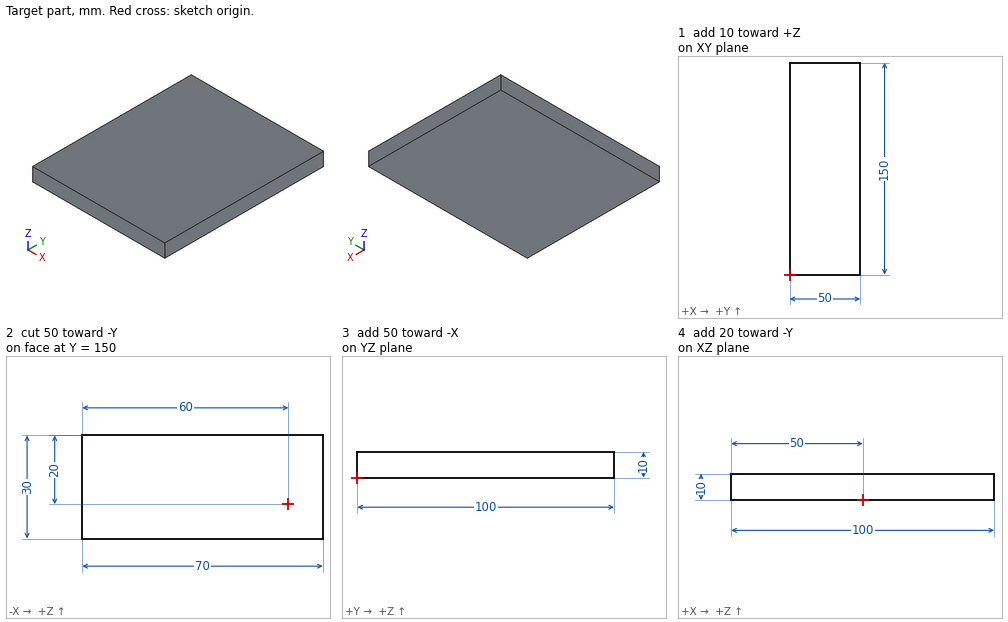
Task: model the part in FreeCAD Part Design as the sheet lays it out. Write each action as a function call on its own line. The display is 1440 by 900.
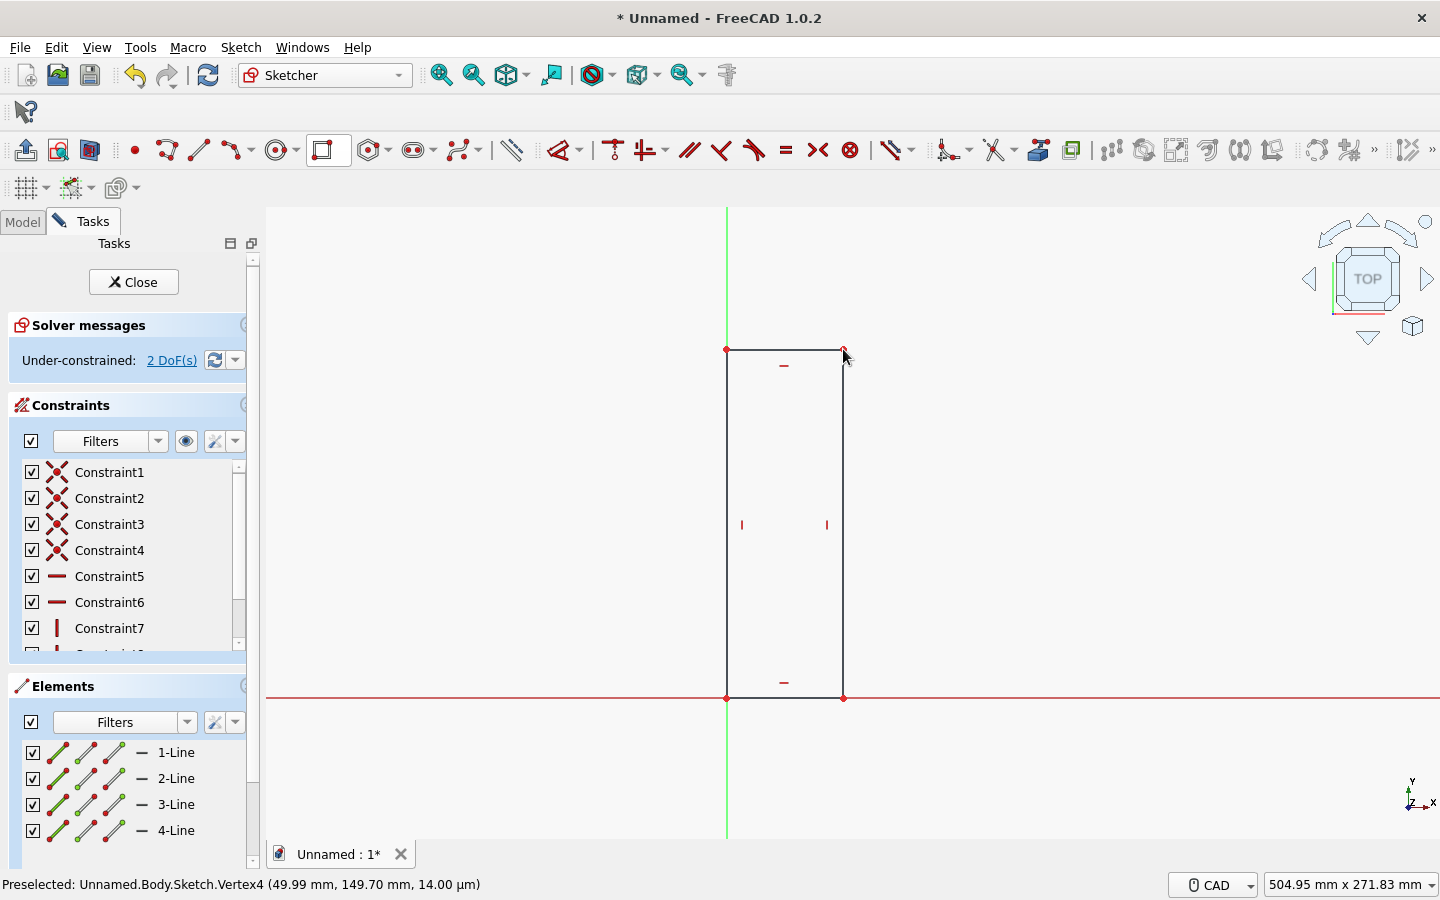
click(558, 150)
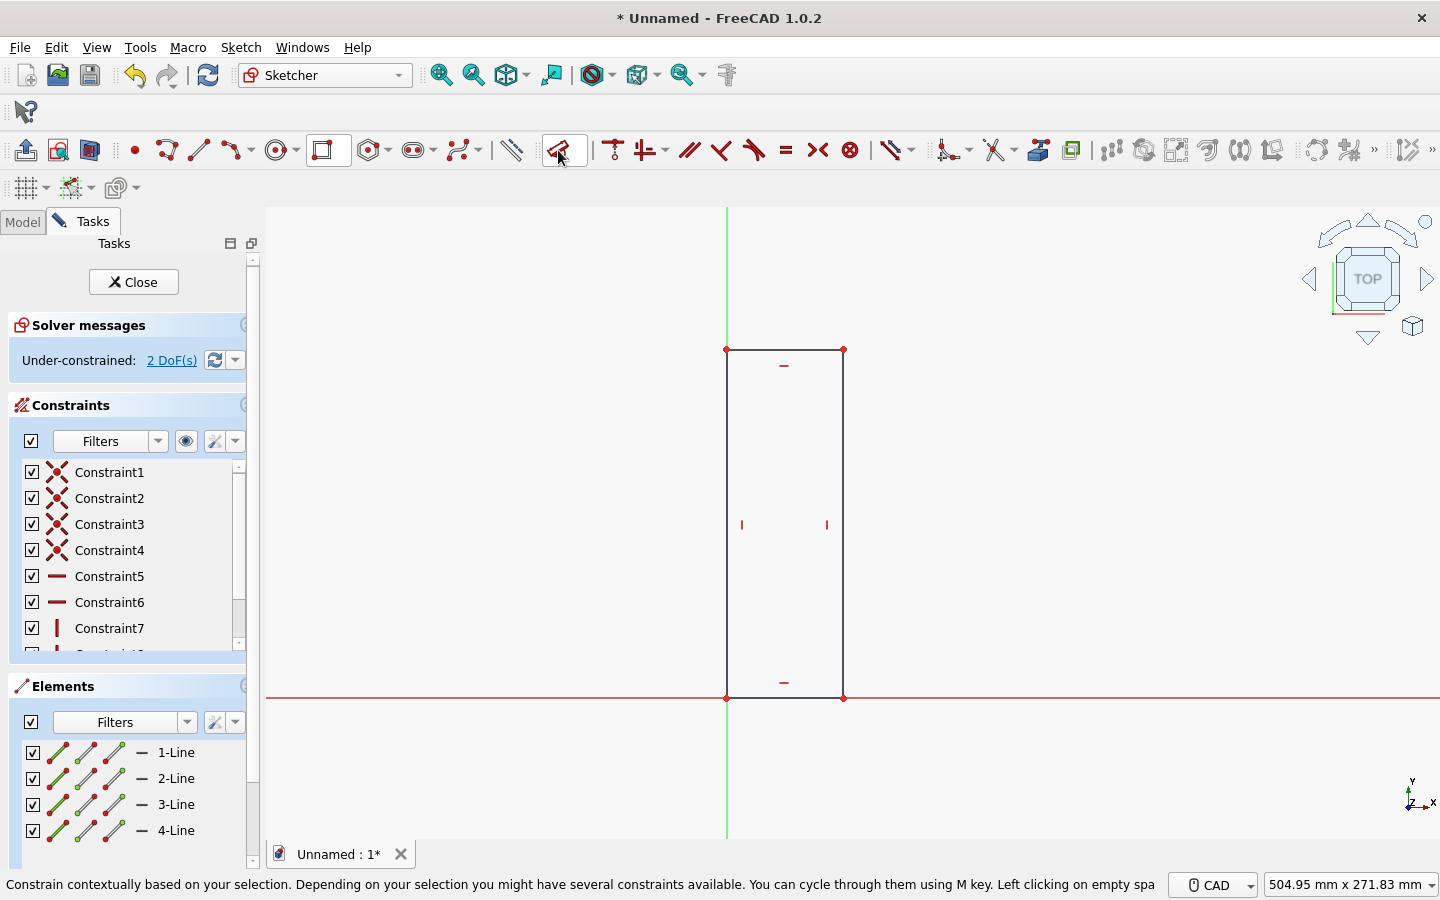
click(762, 698)
click(785, 732)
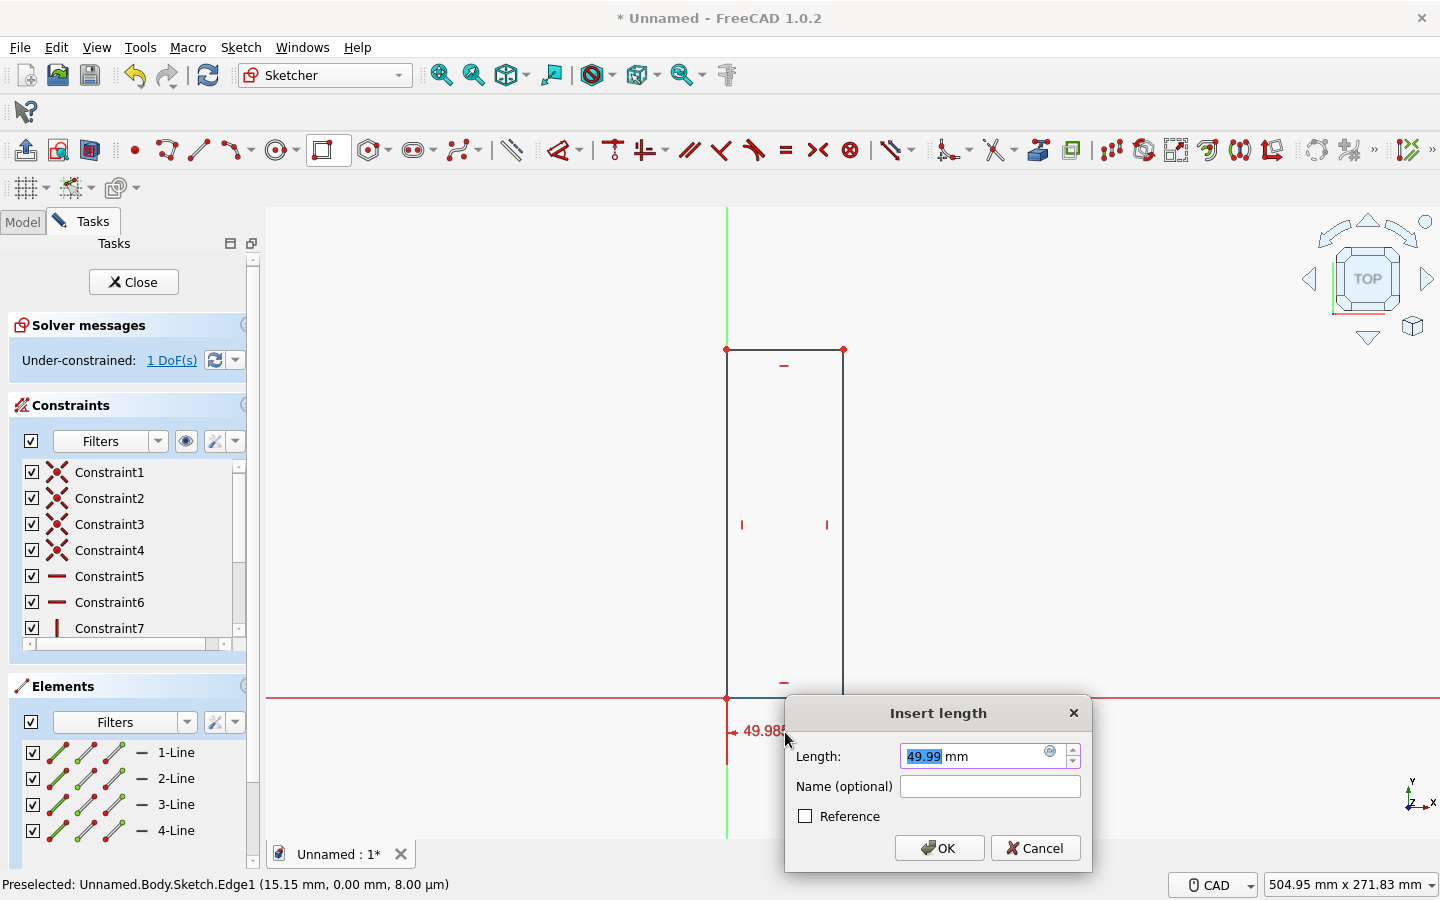
text(50)
key(Return)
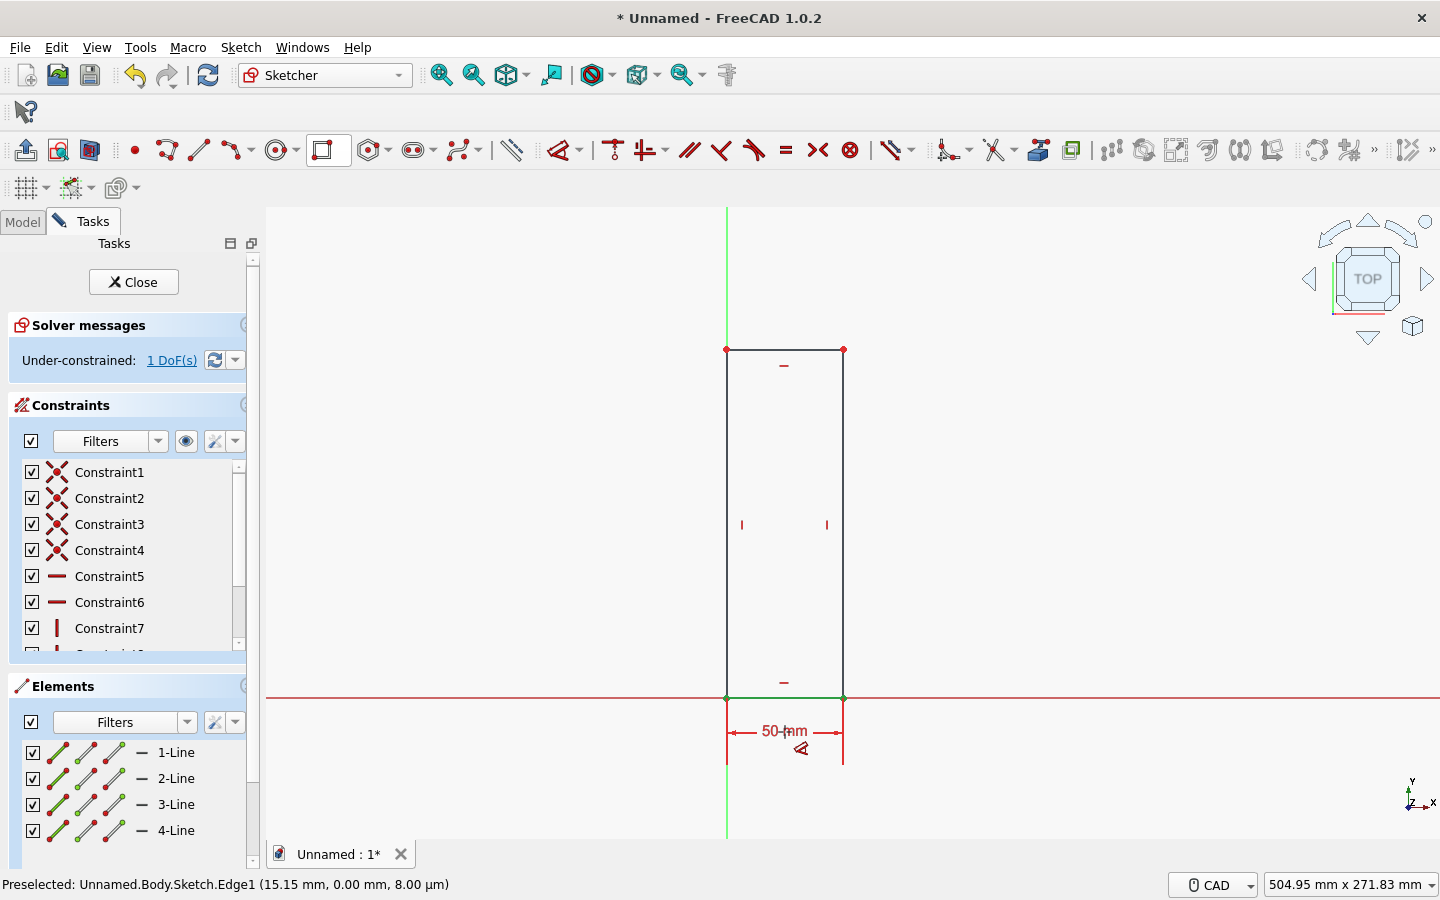
click(843, 594)
click(877, 524)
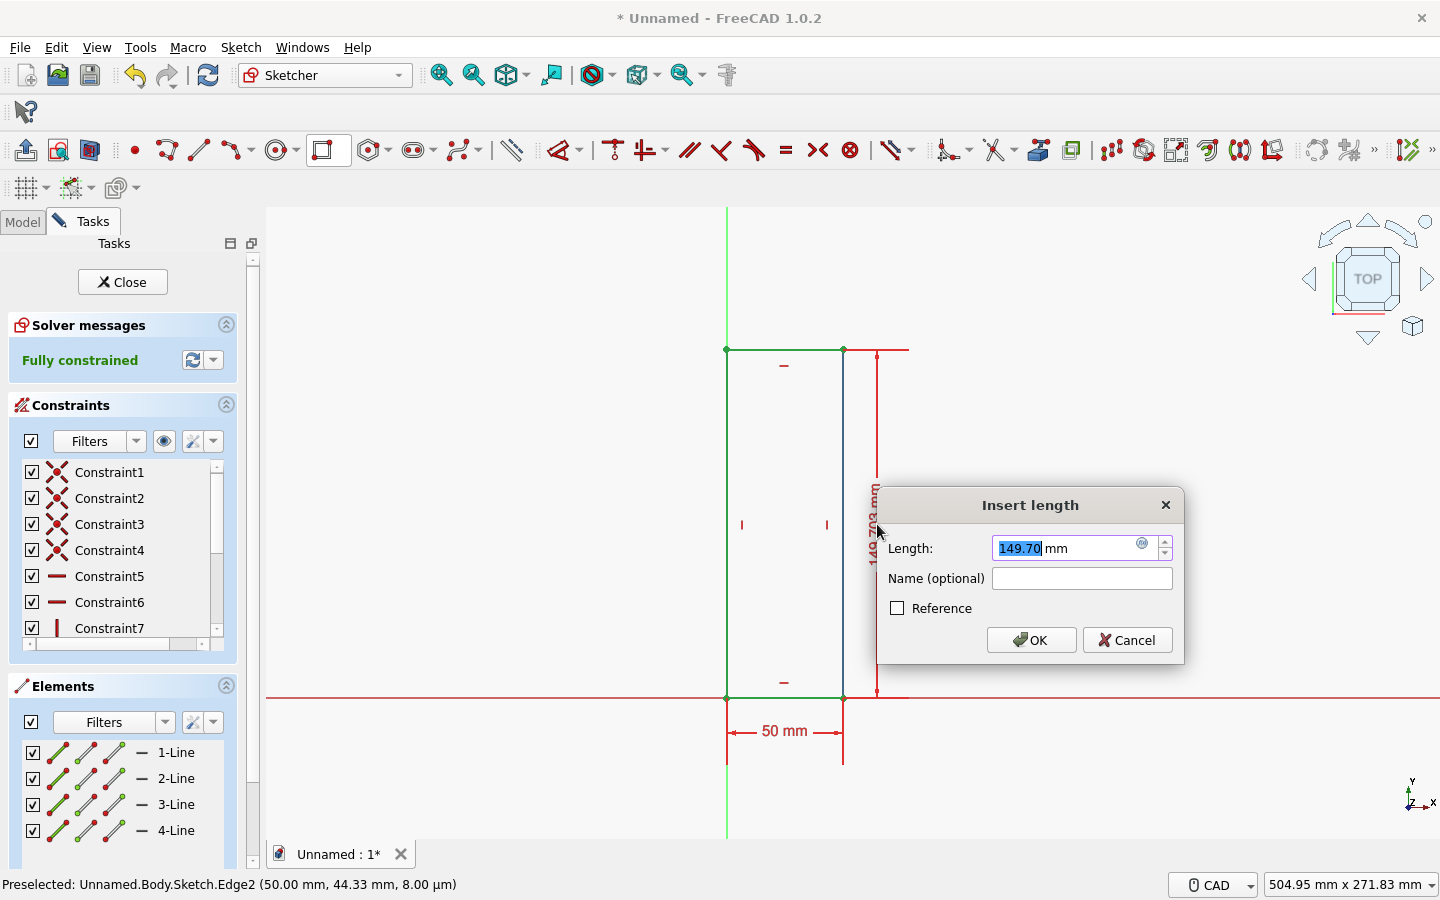
text(150)
key(Return)
key(Escape)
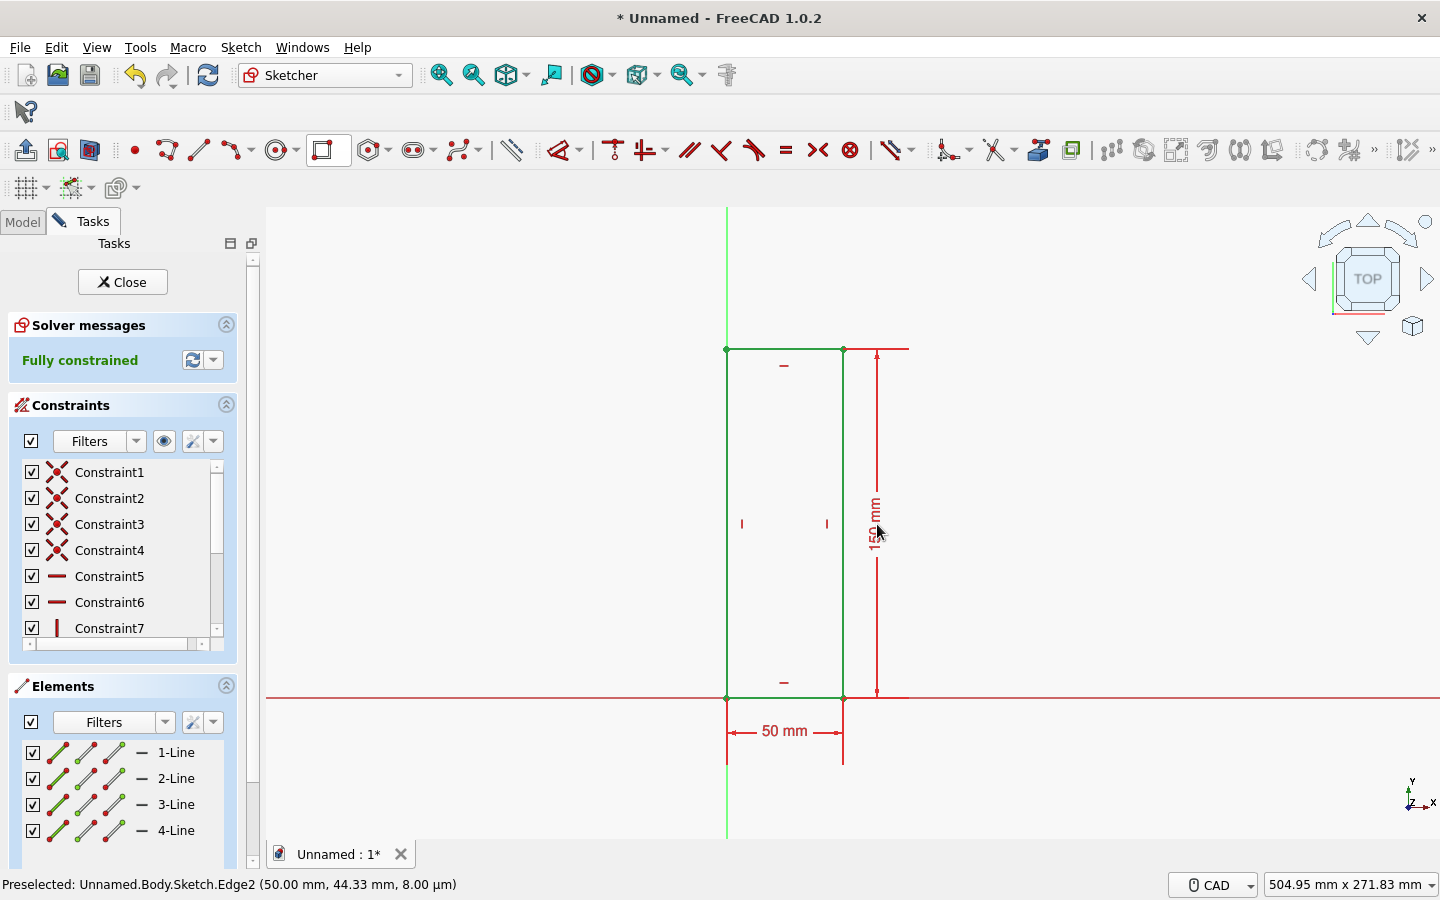
click(123, 282)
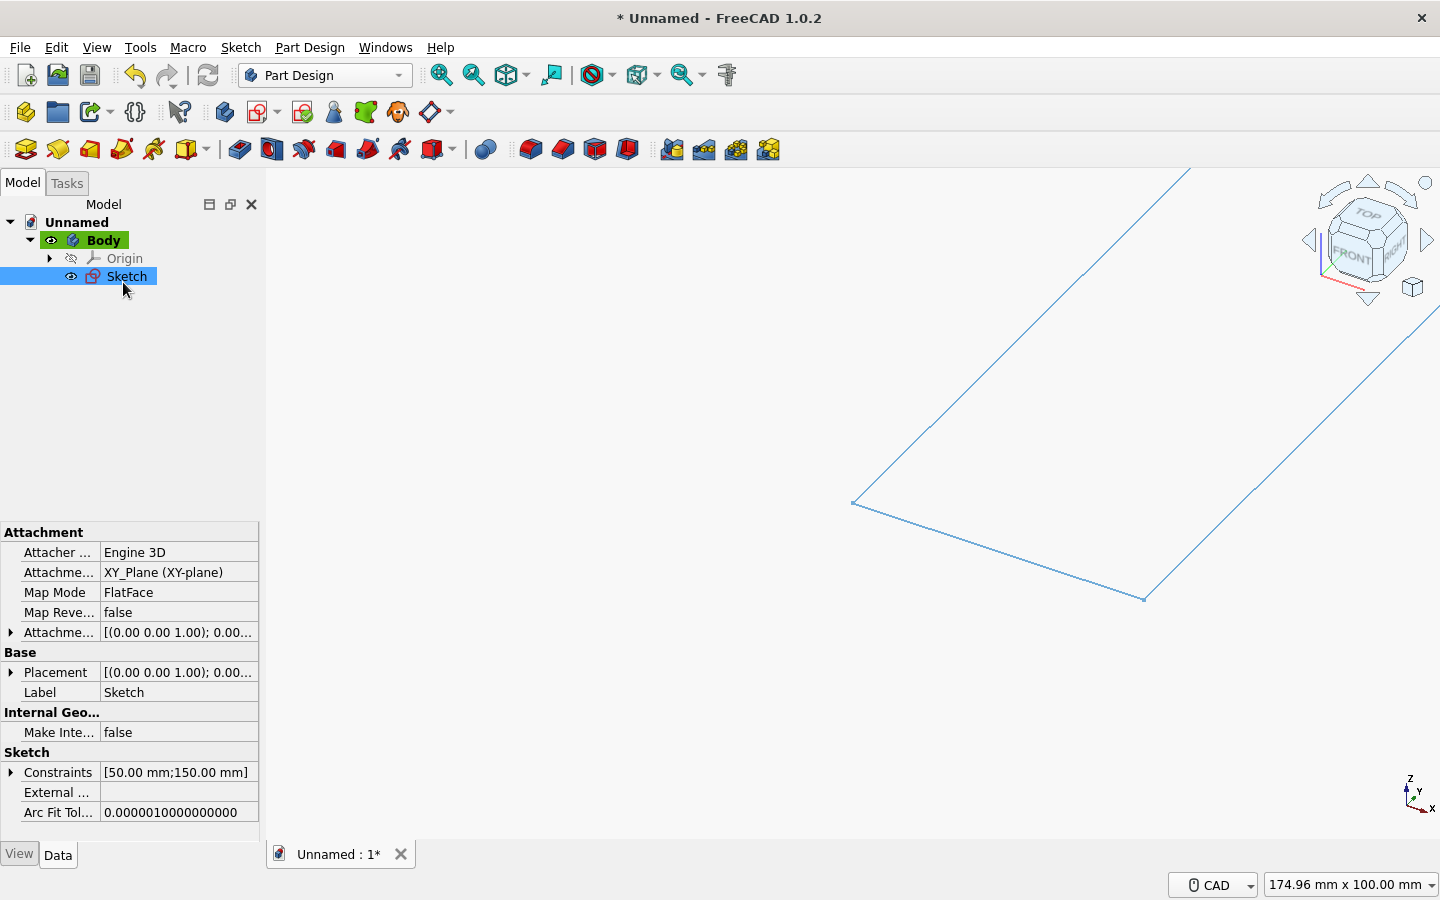
click(26, 150)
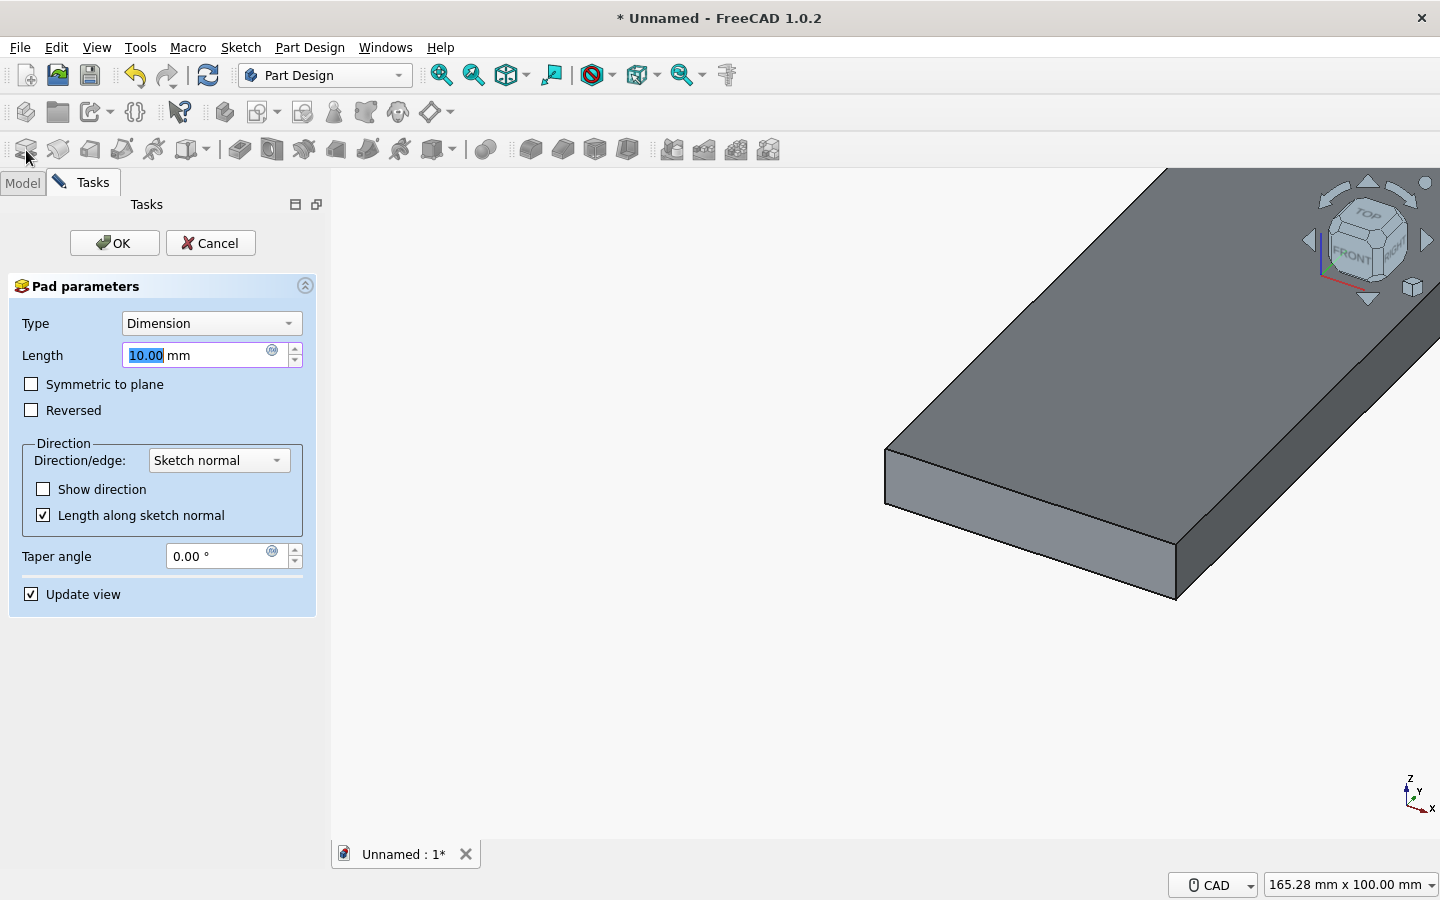
text(10)
key(Tab)